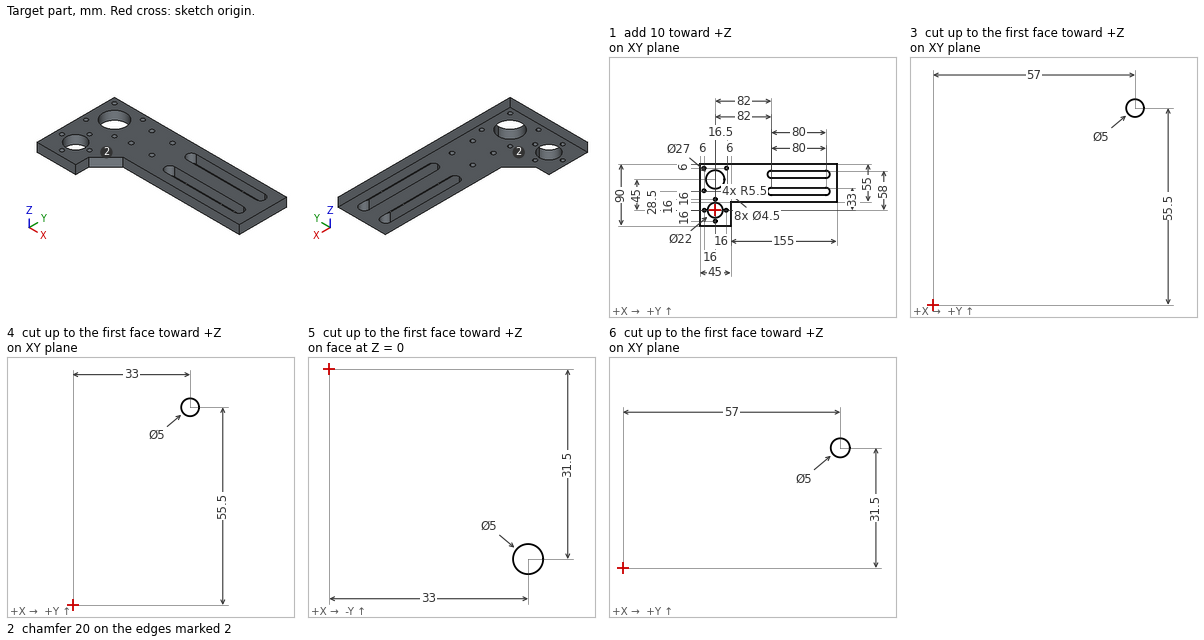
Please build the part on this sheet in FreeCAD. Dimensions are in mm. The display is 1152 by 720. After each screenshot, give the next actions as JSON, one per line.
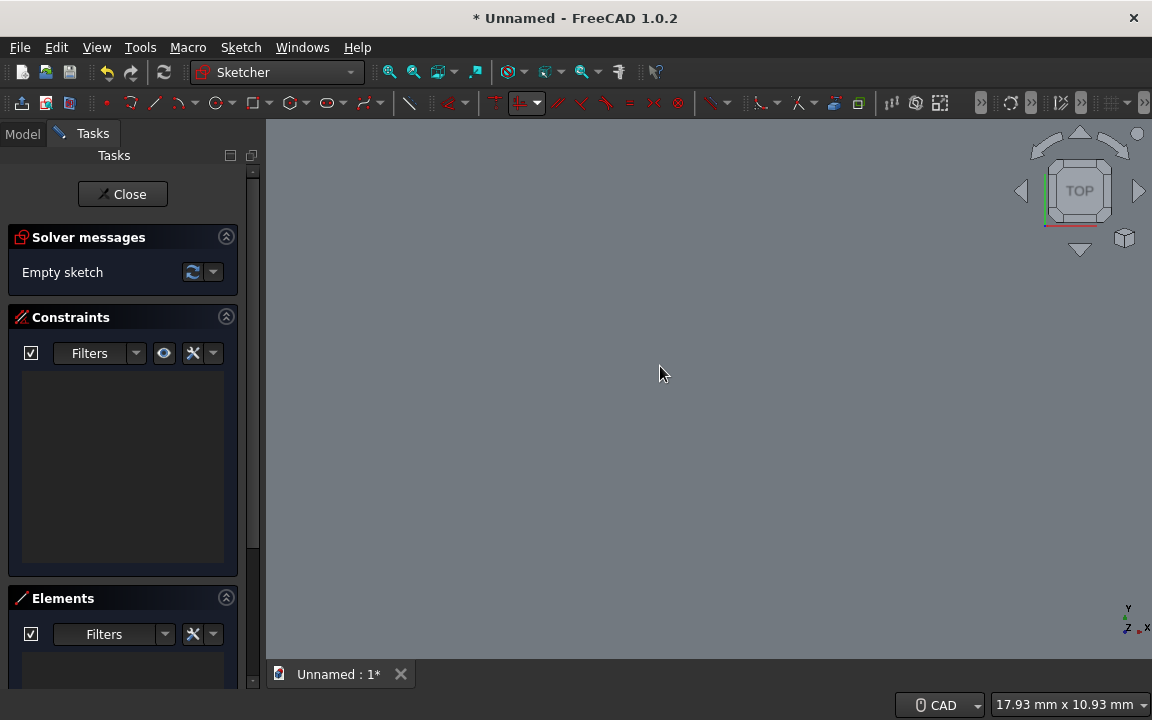
{"action": "scroll", "coordinate": [587, 345], "scroll_direction": "up", "scroll_amount": 2}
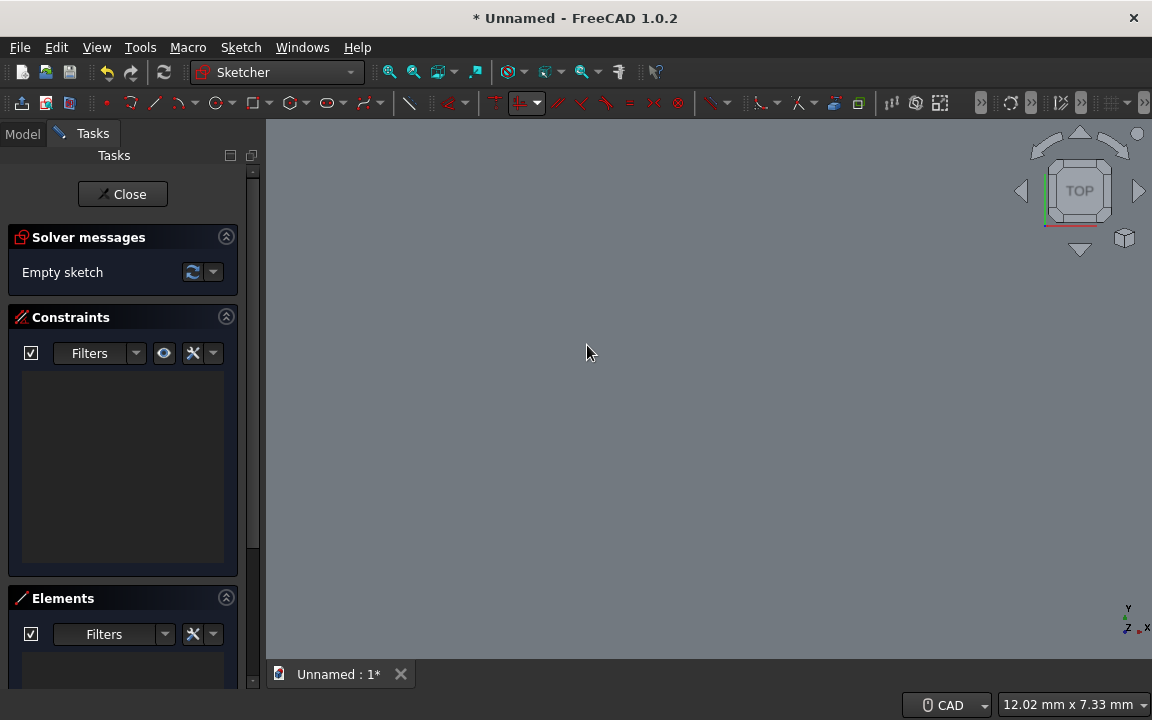
{"action": "left_click", "coordinate": [216, 104]}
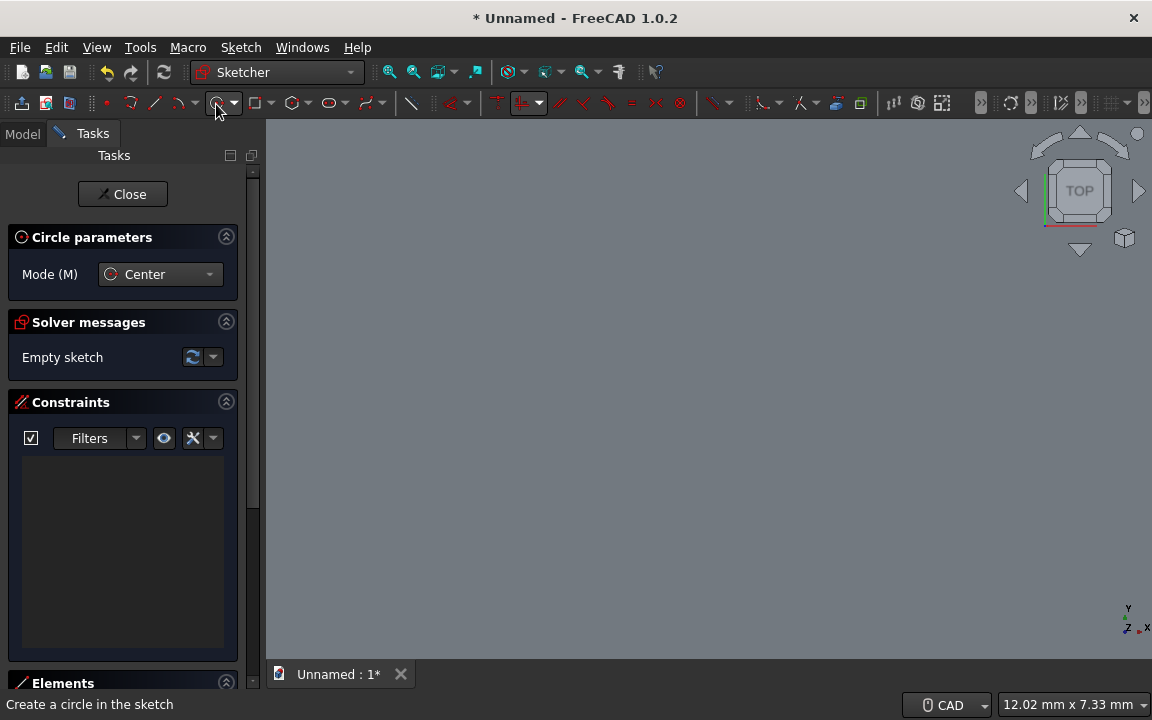
{"action": "left_click", "coordinate": [640, 389]}
{"action": "mouse_move", "coordinate": [771, 259]}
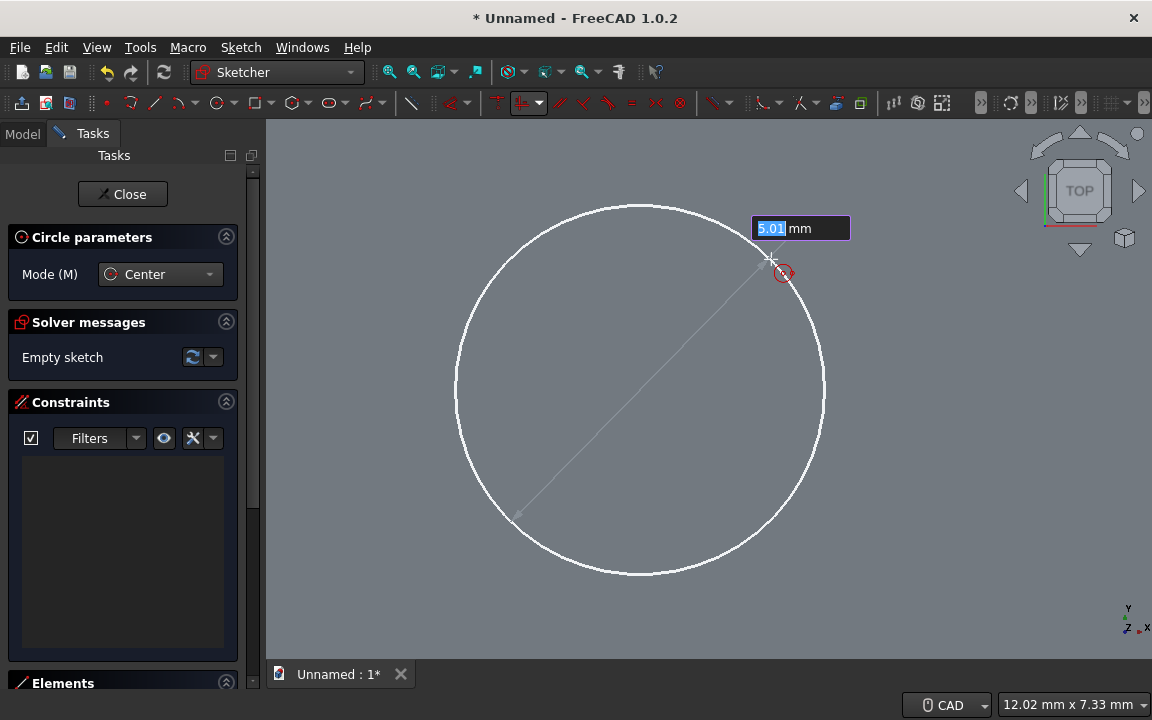
{"action": "type", "text": "5"}
{"action": "key", "text": "Return"}
{"action": "key", "text": "Escape"}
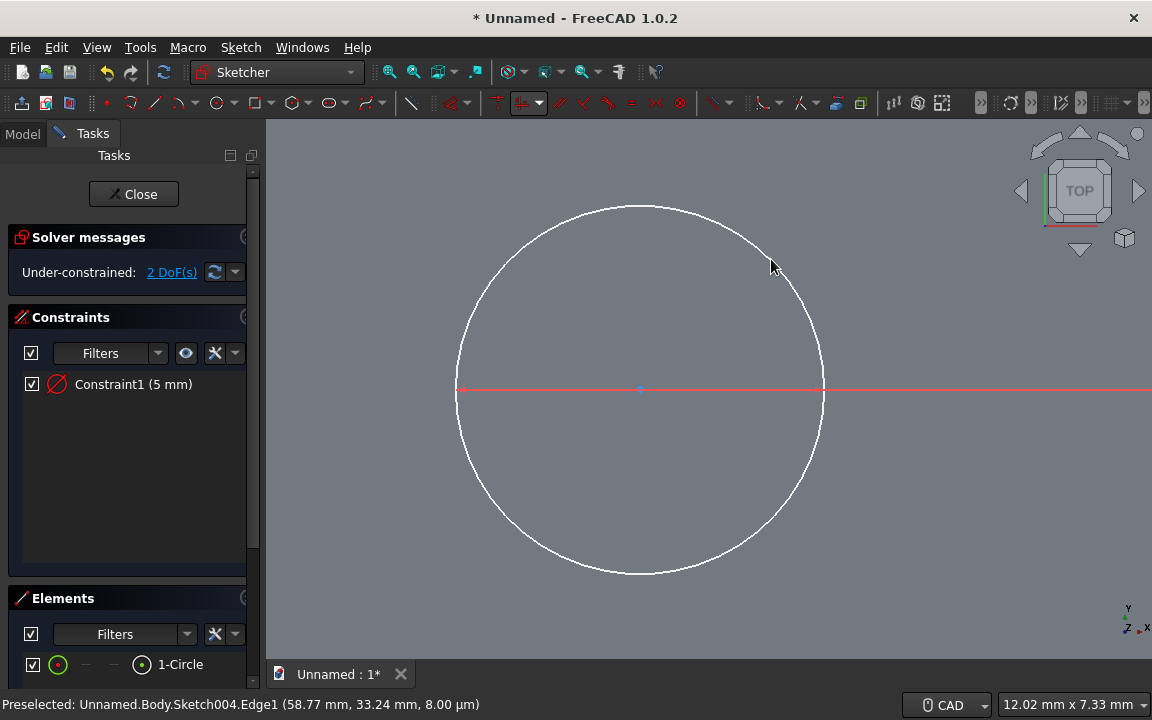
{"action": "key", "text": "d"}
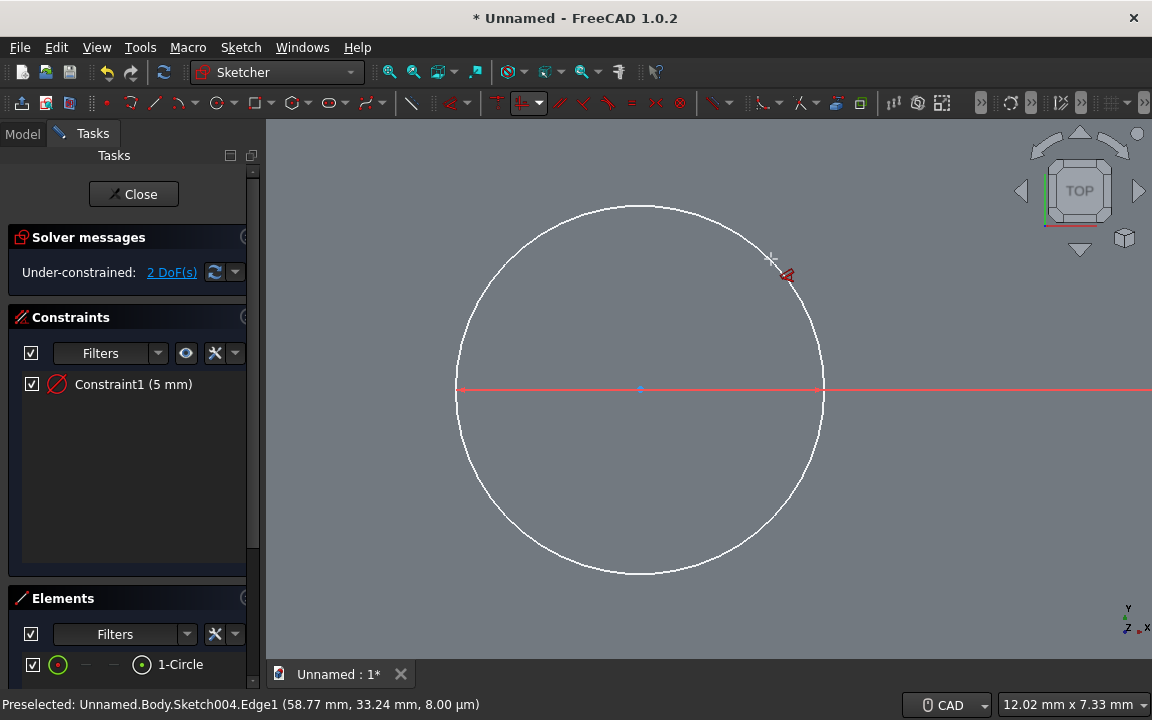
{"action": "left_click", "coordinate": [640, 390]}
{"action": "left_click", "coordinate": [387, 356]}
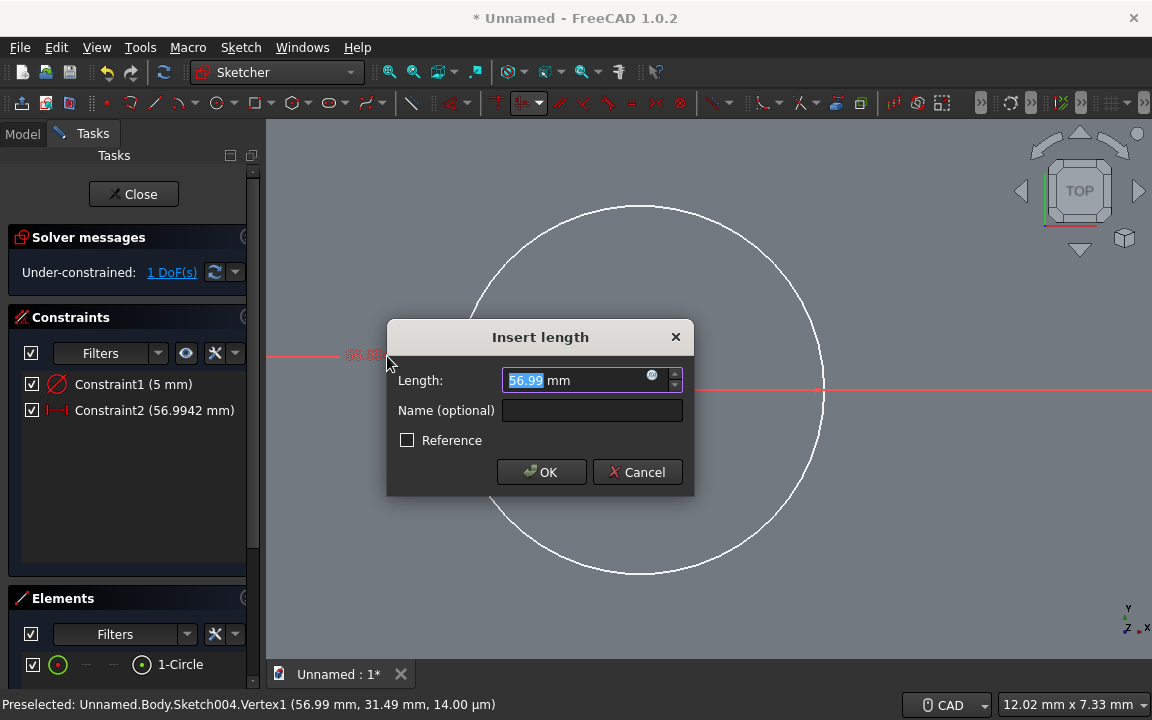
{"action": "type", "text": "57"}
{"action": "key", "text": "Return"}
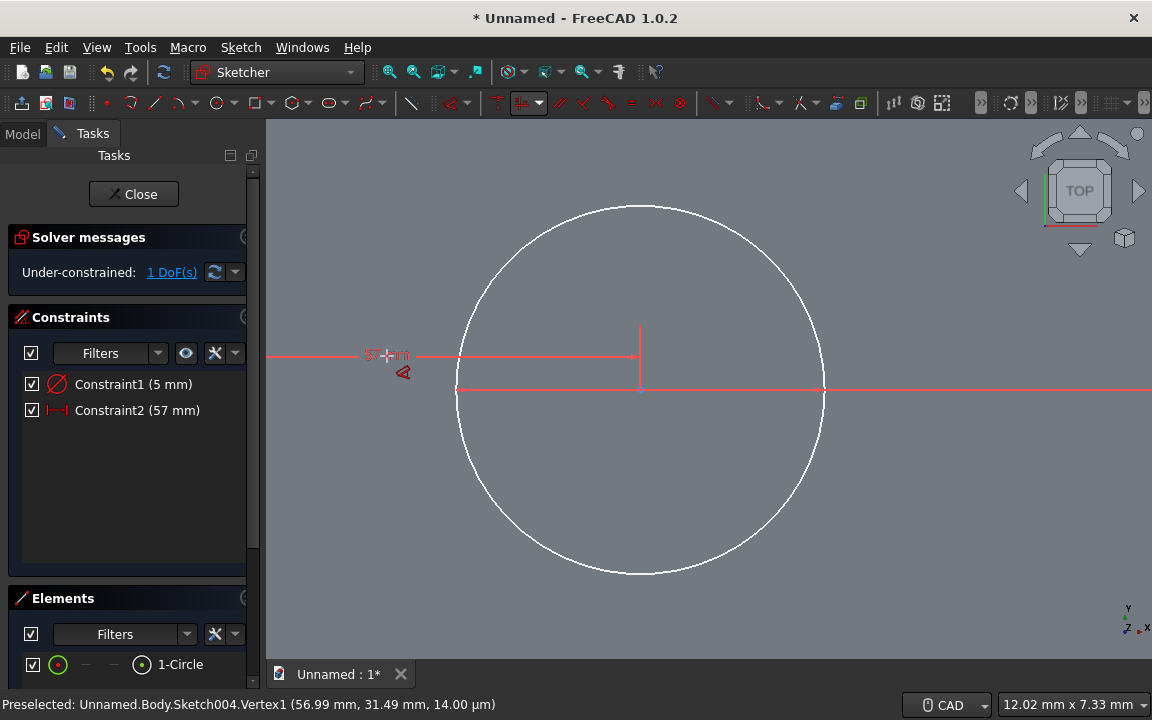
{"action": "left_click", "coordinate": [640, 390]}
{"action": "left_click", "coordinate": [674, 511]}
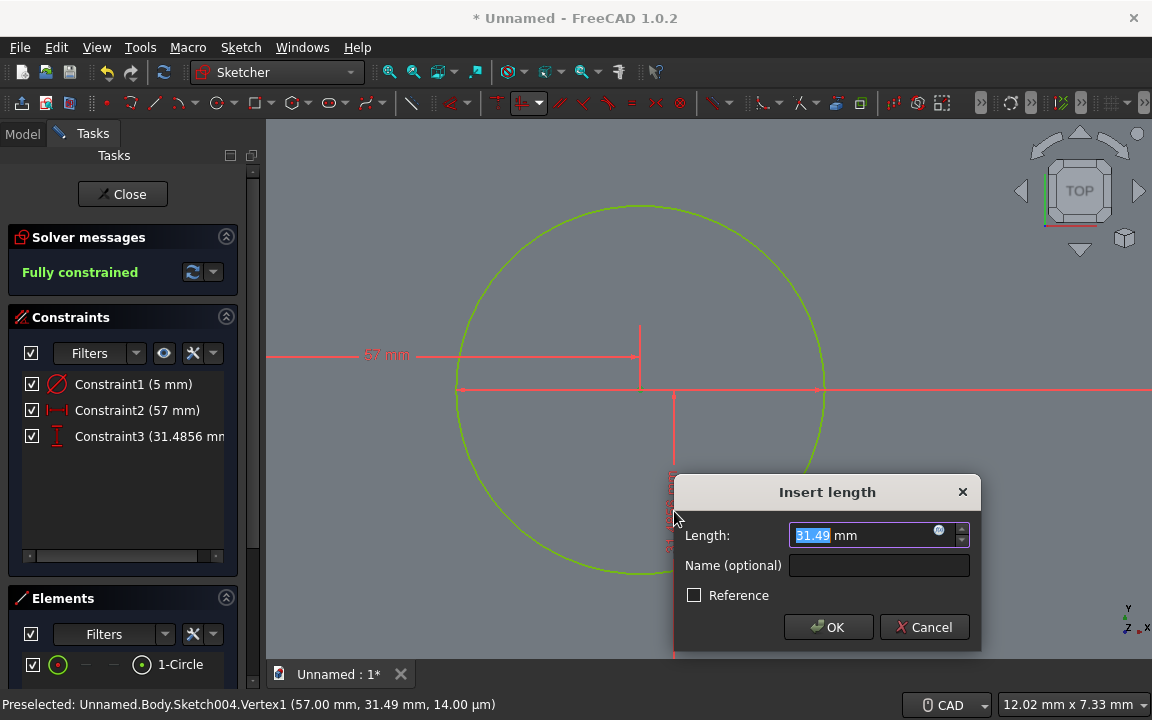
{"action": "type", "text": "31.5"}
{"action": "key", "text": "Return"}
{"action": "key", "text": "Escape"}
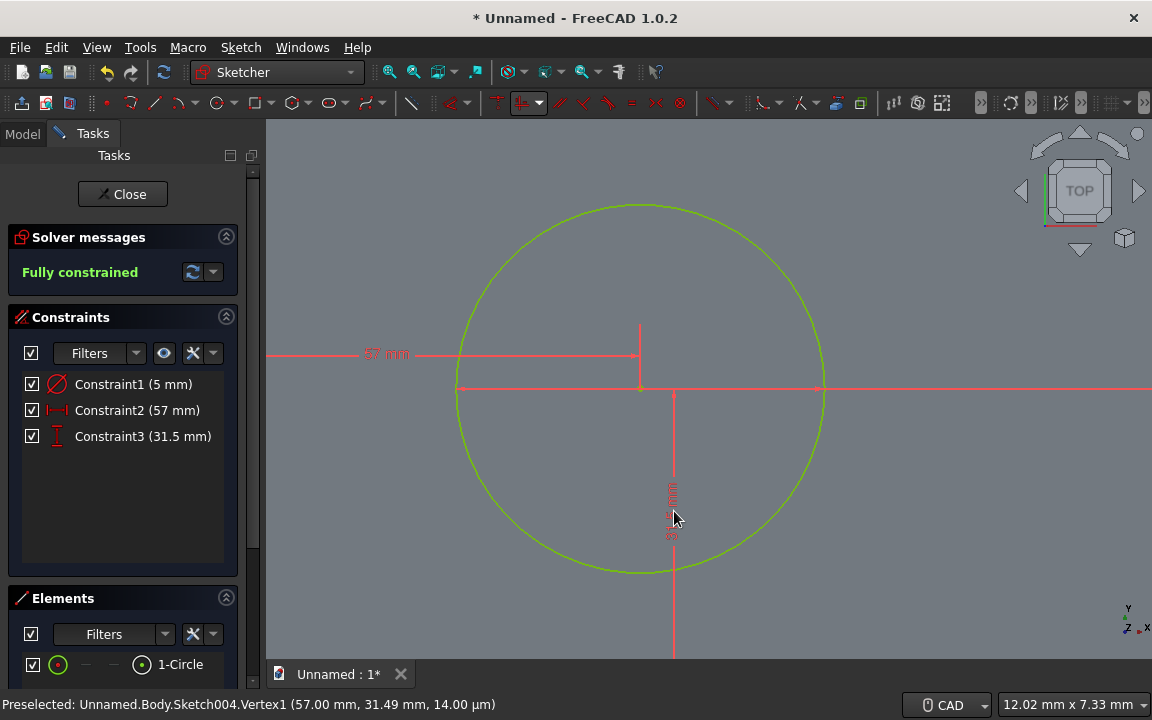
{"action": "left_click", "coordinate": [123, 194]}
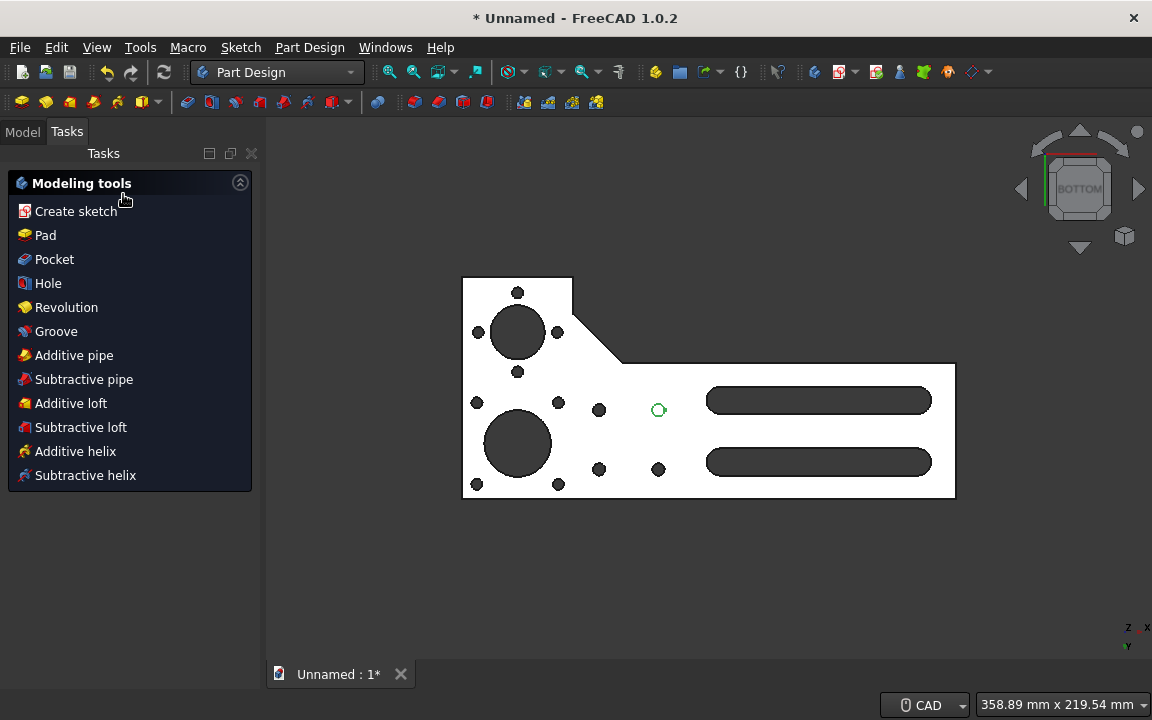
{"action": "left_click", "coordinate": [188, 102]}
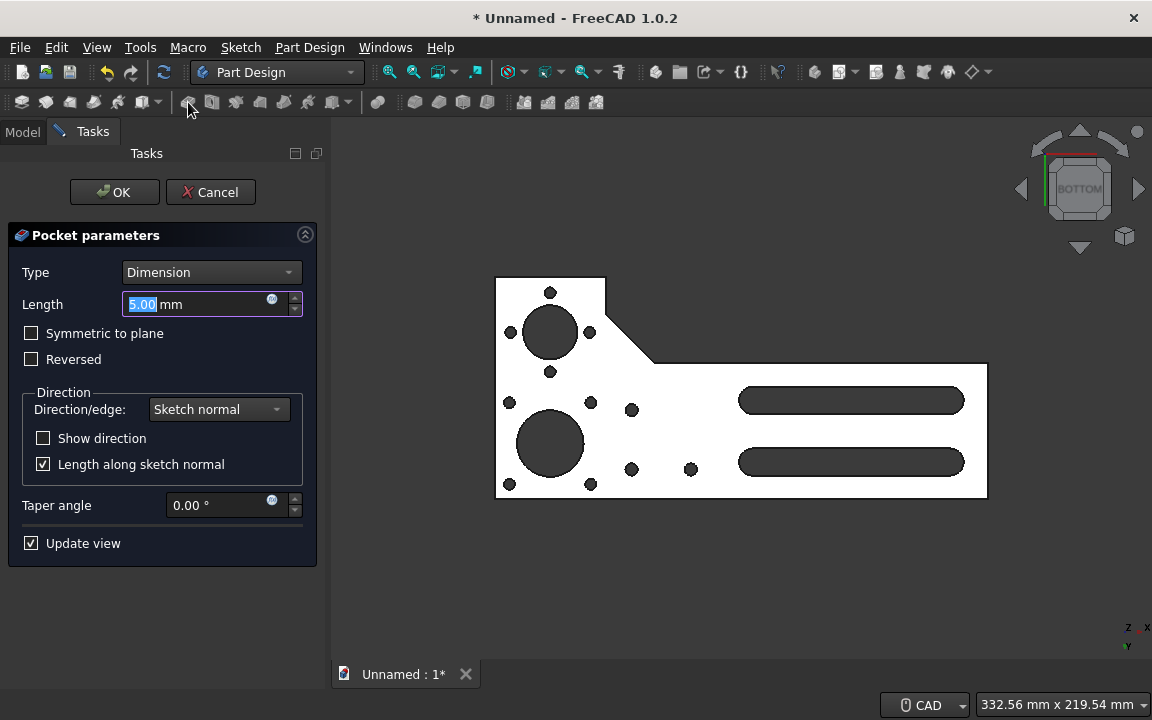
{"action": "left_click", "coordinate": [212, 272]}